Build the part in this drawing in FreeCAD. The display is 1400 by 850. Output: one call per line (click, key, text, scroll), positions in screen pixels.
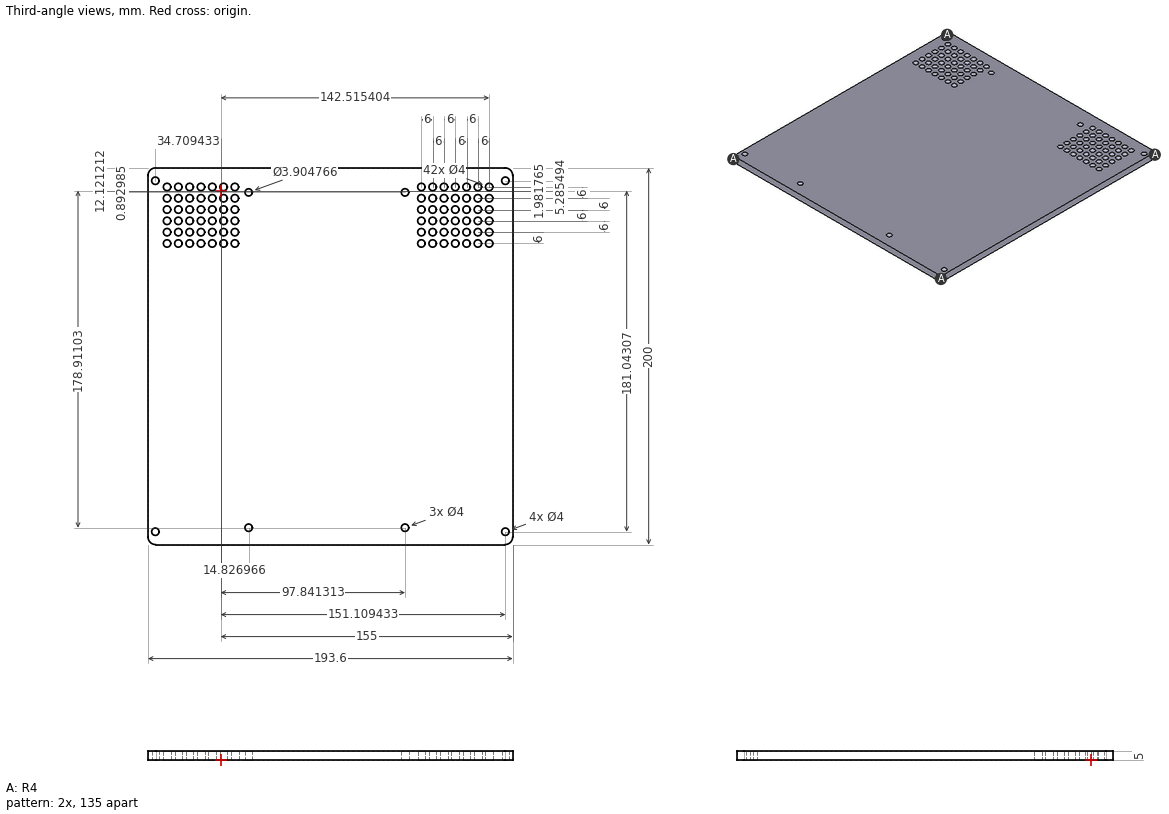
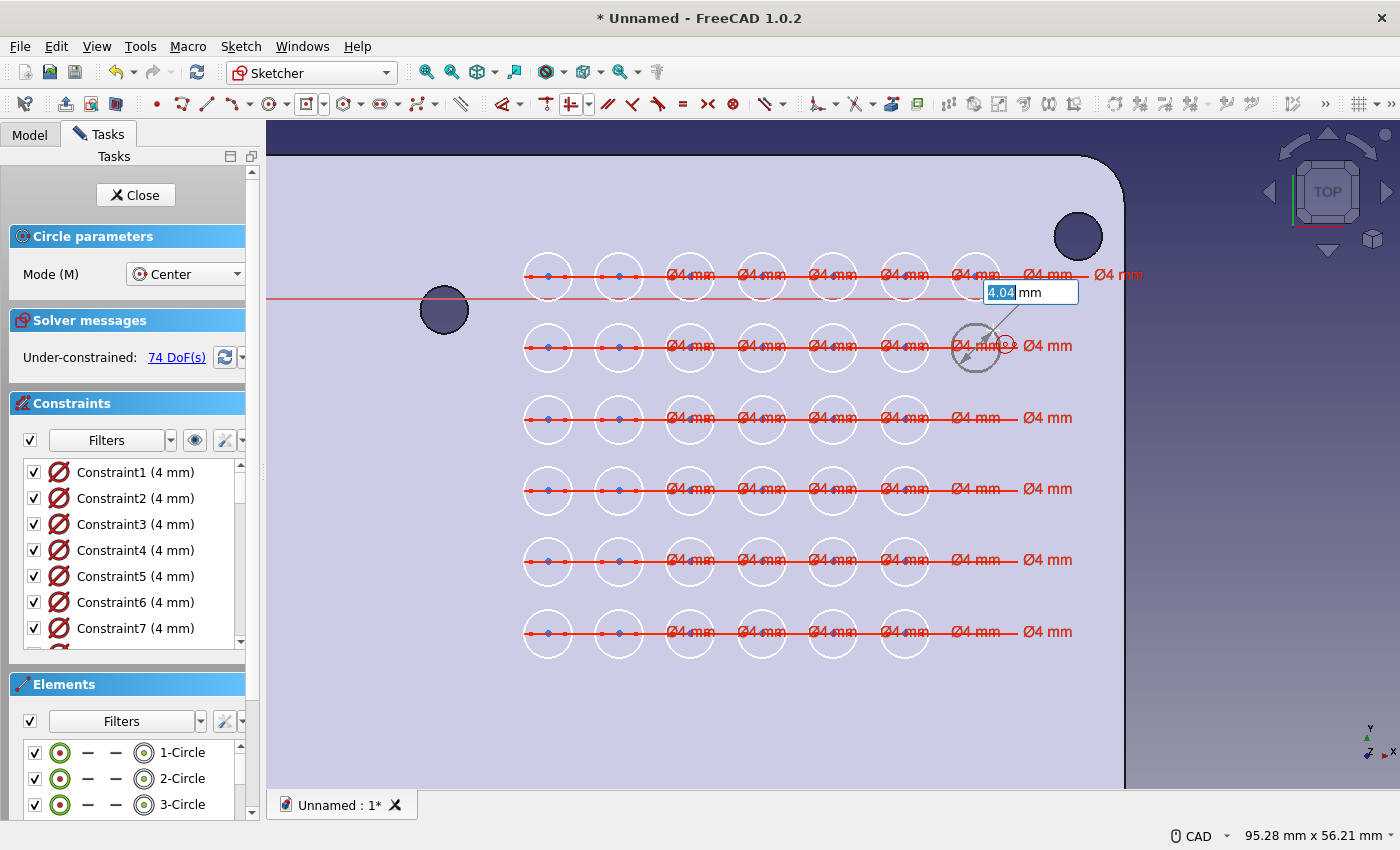
text(4)
key(Return)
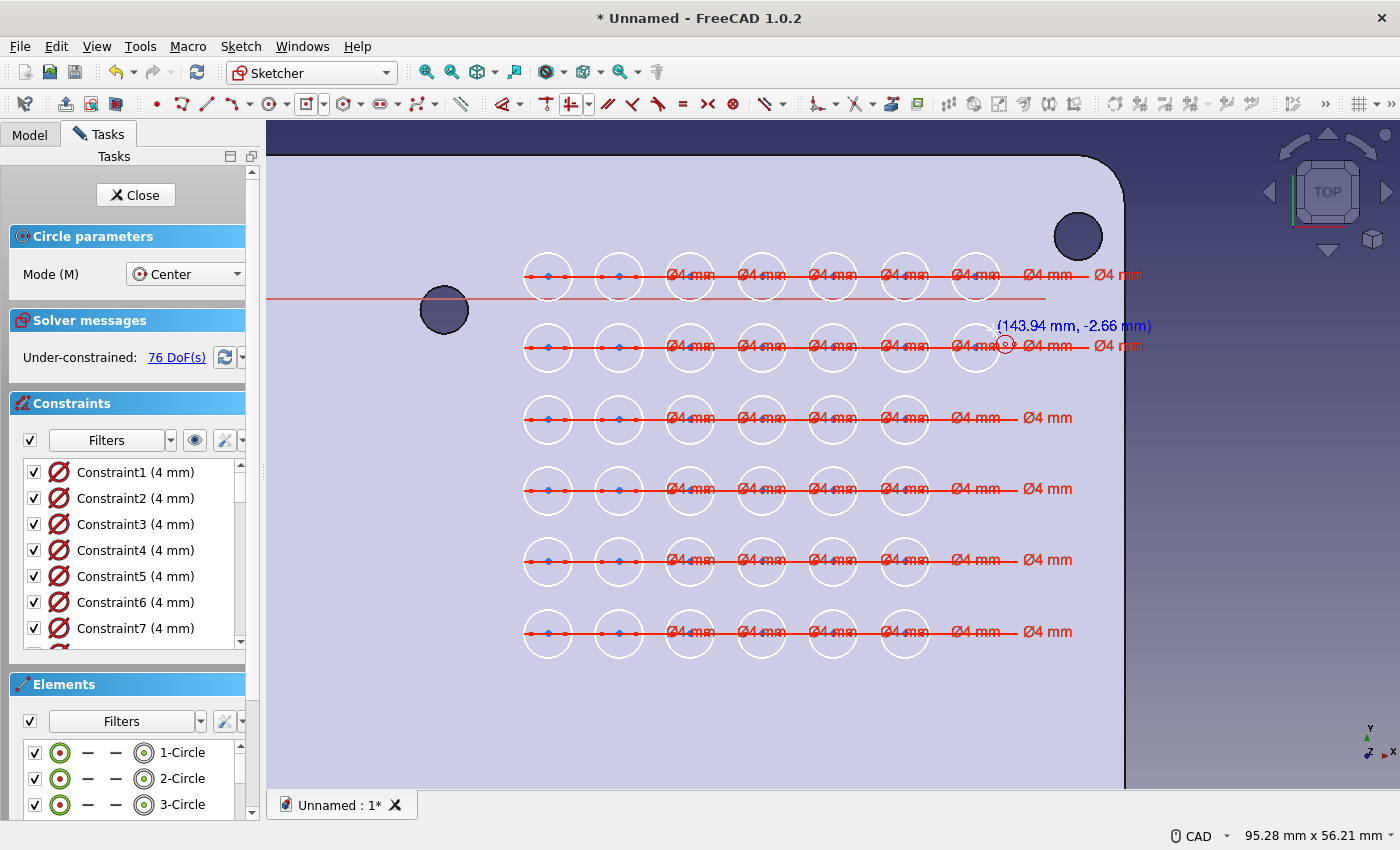
click(976, 419)
move(993, 402)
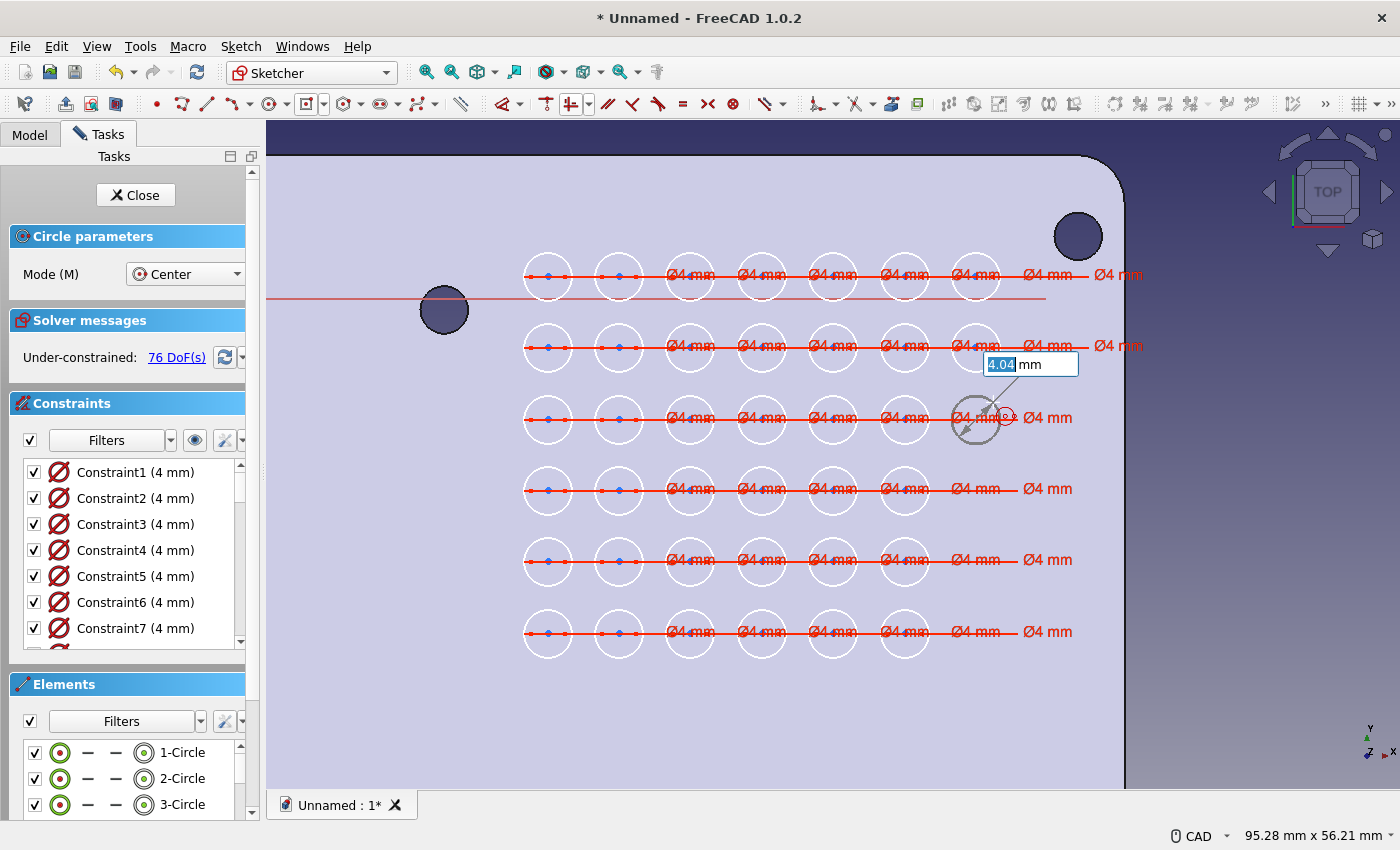
text(4)
key(Return)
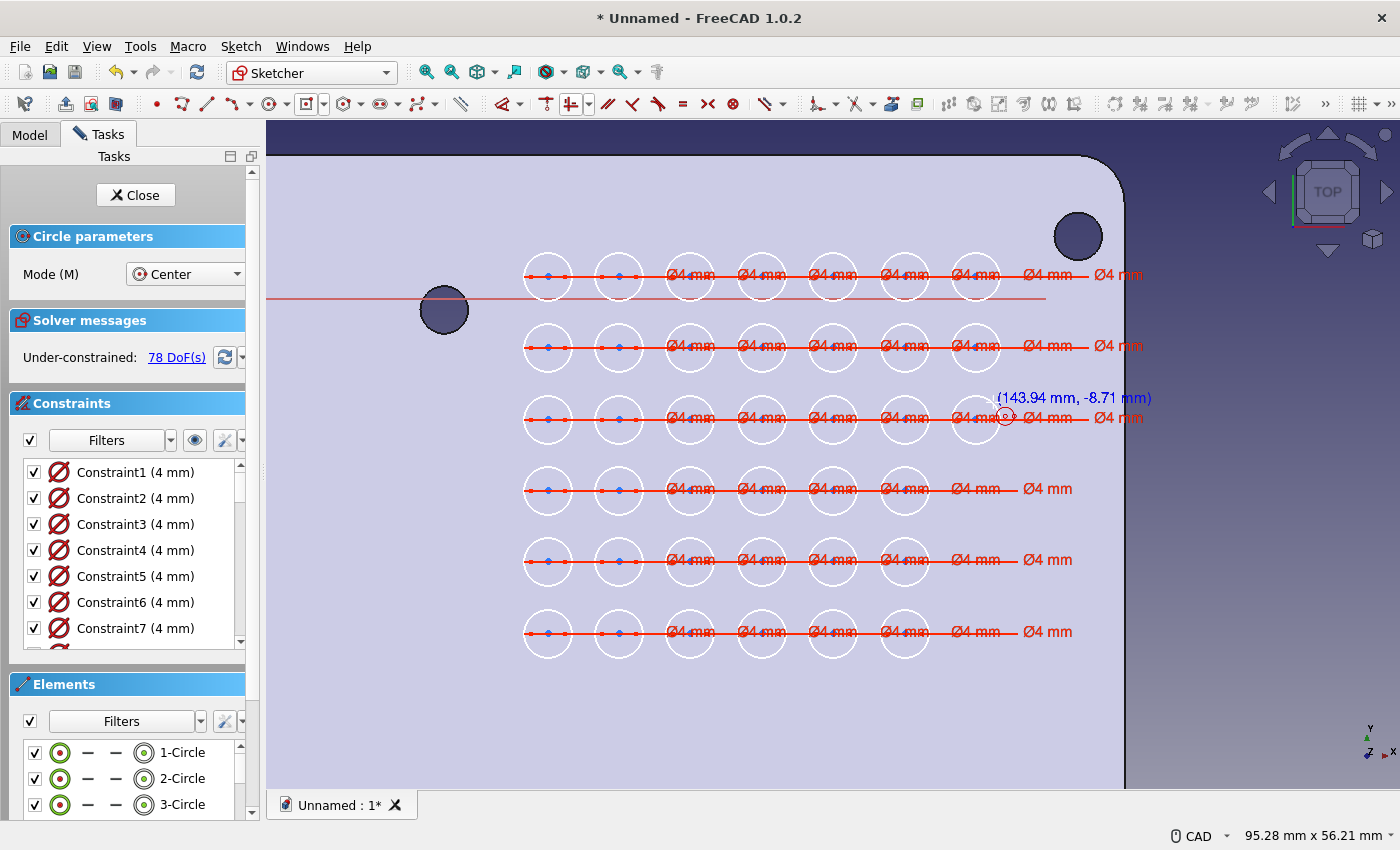
click(976, 490)
move(993, 473)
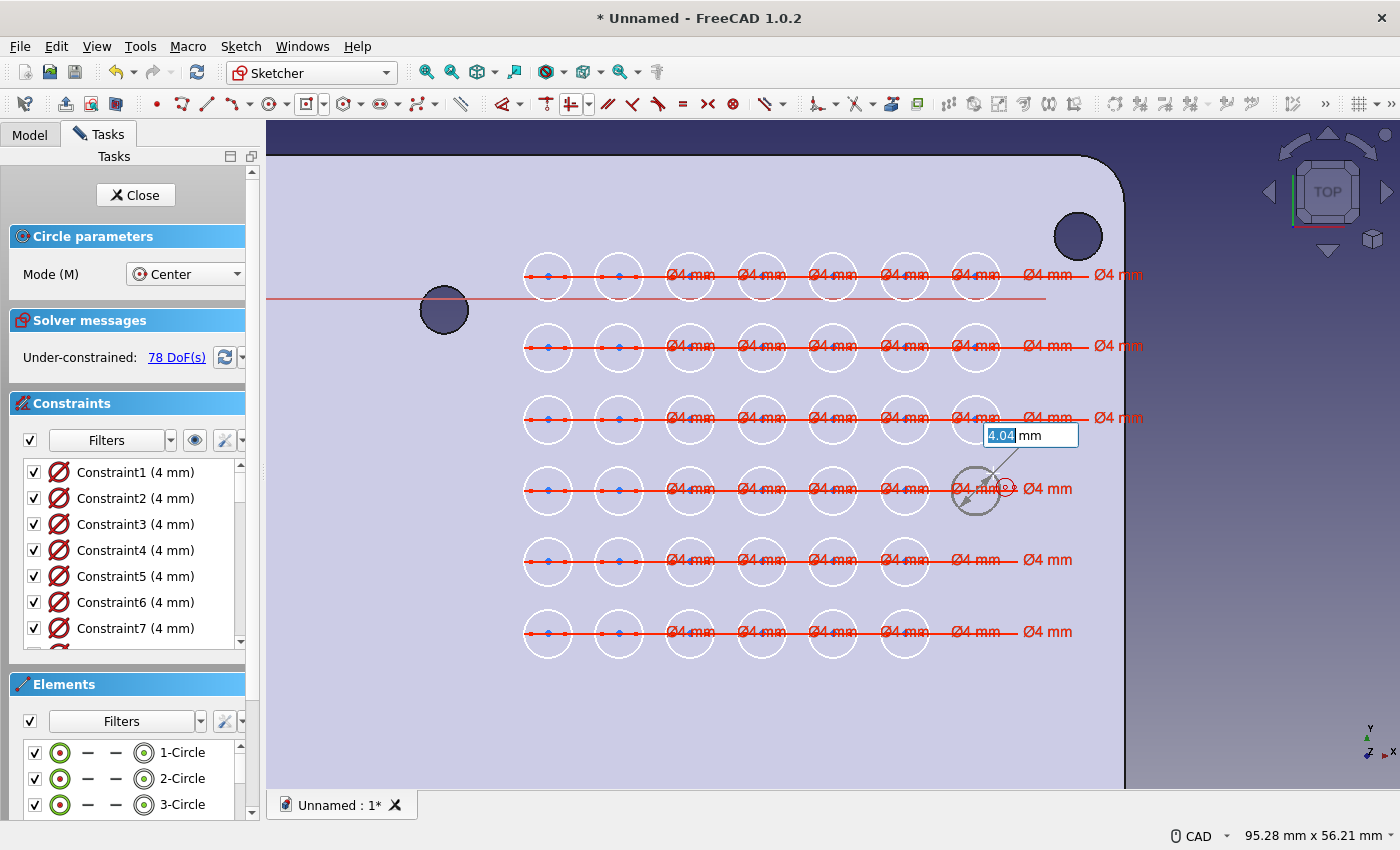
text(4)
key(Return)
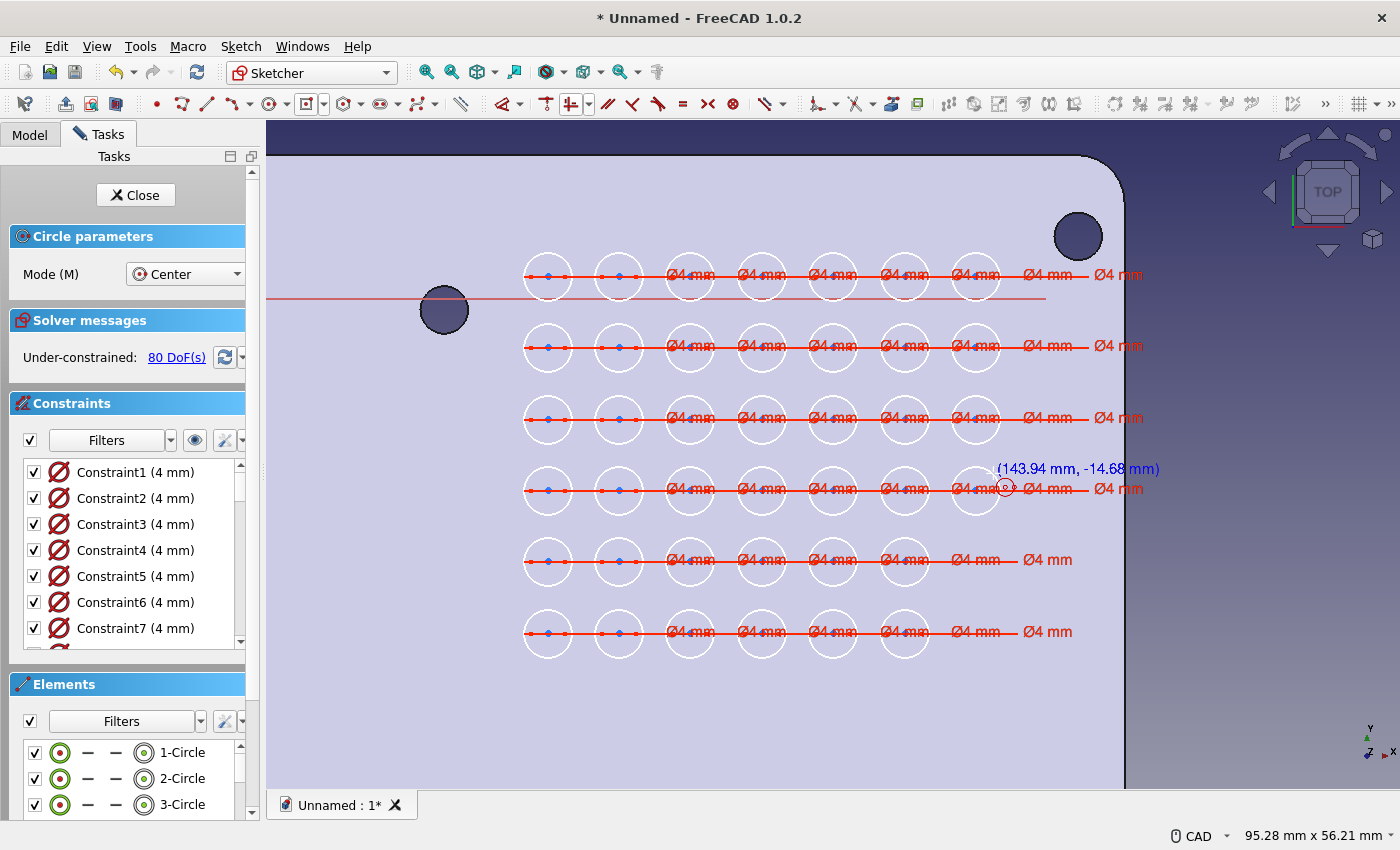
click(976, 561)
move(993, 545)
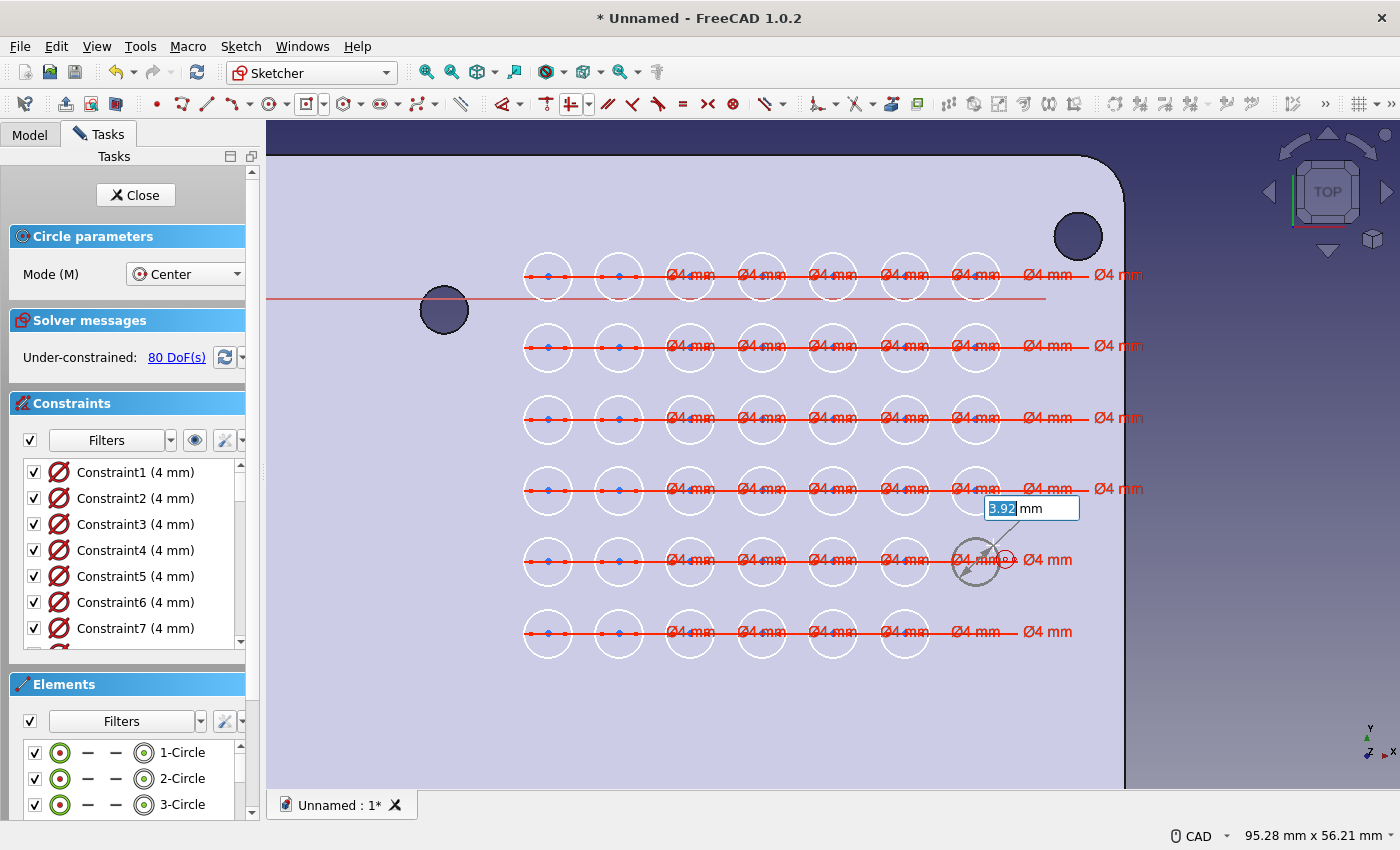
text(4)
key(Return)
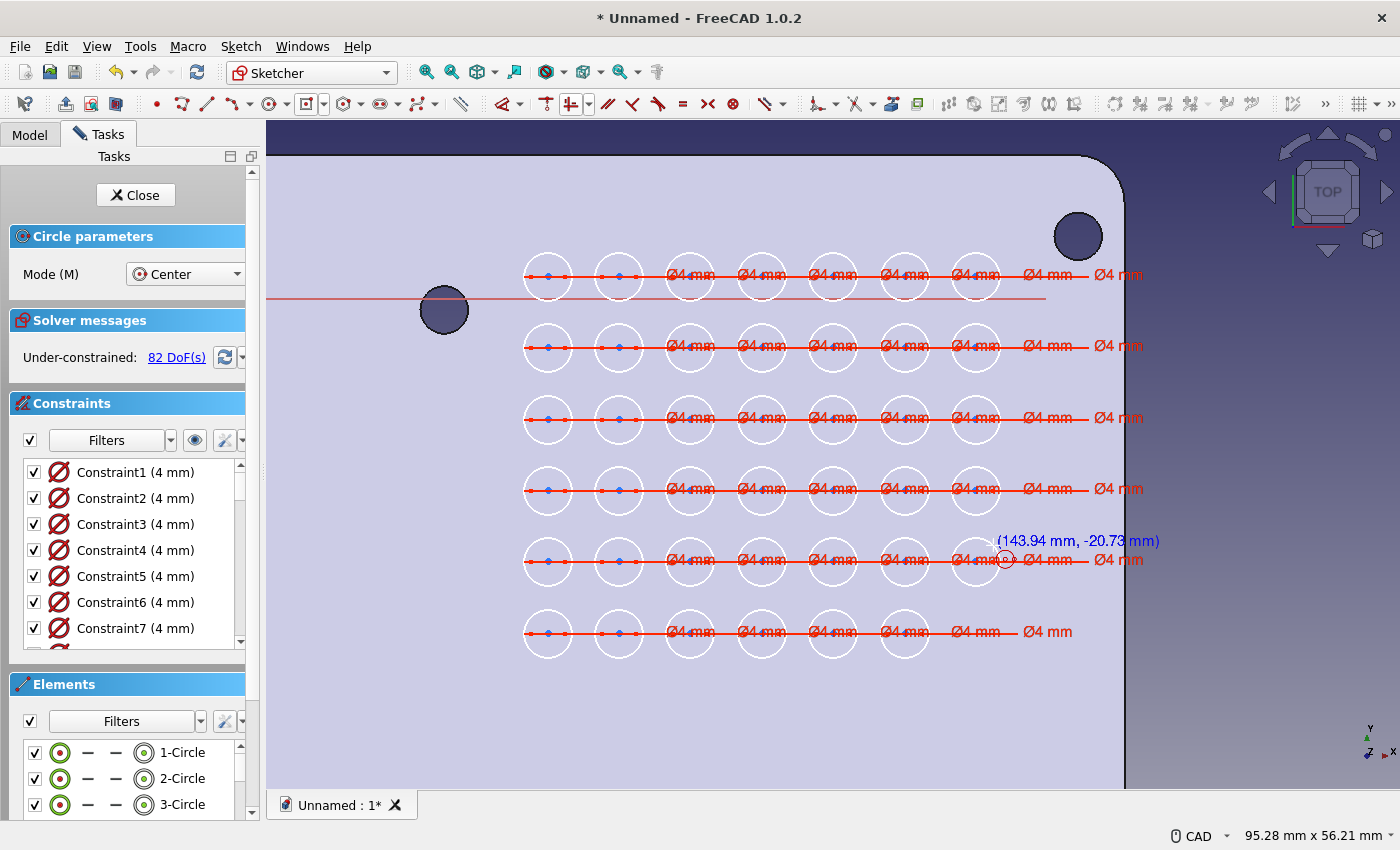
click(976, 633)
move(993, 616)